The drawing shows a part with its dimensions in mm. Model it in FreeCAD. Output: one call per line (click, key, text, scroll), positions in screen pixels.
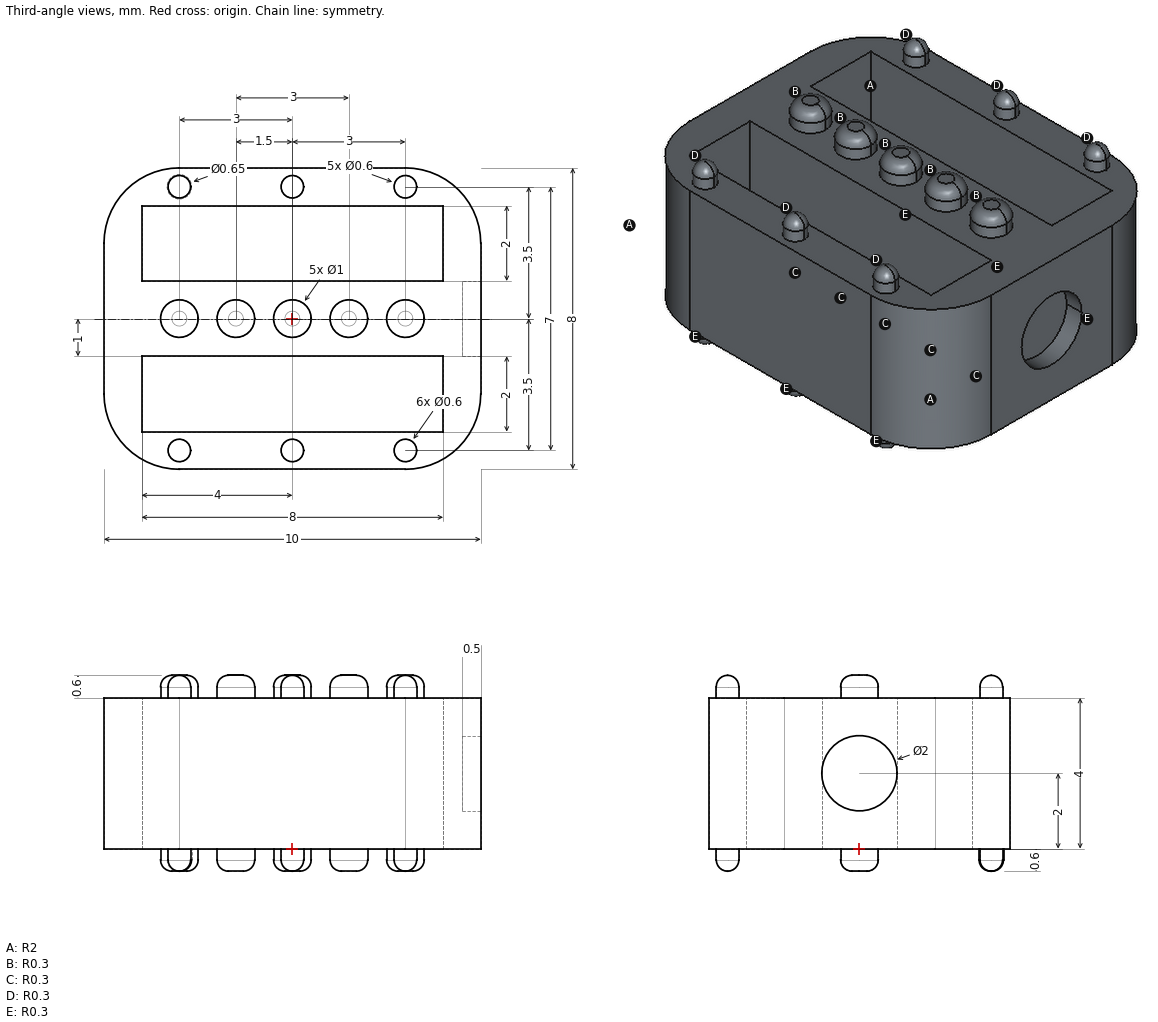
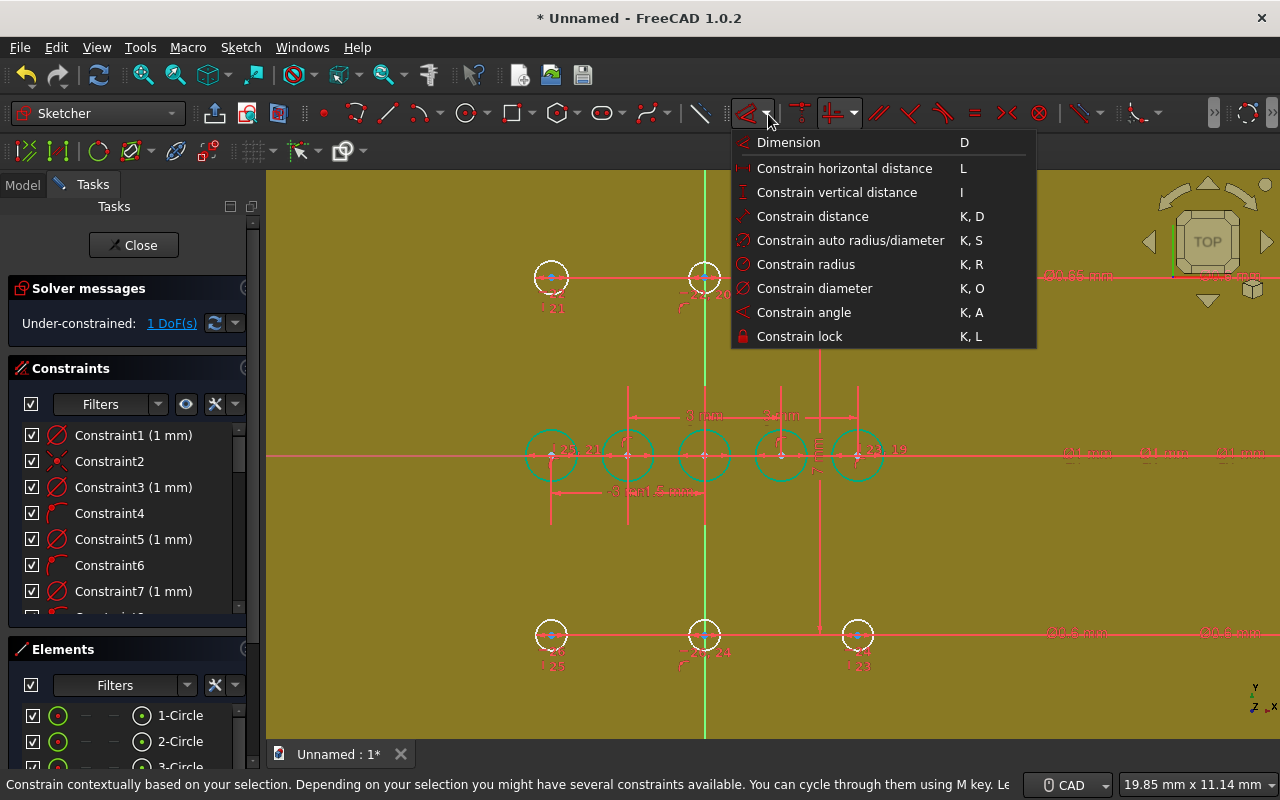
click(884, 192)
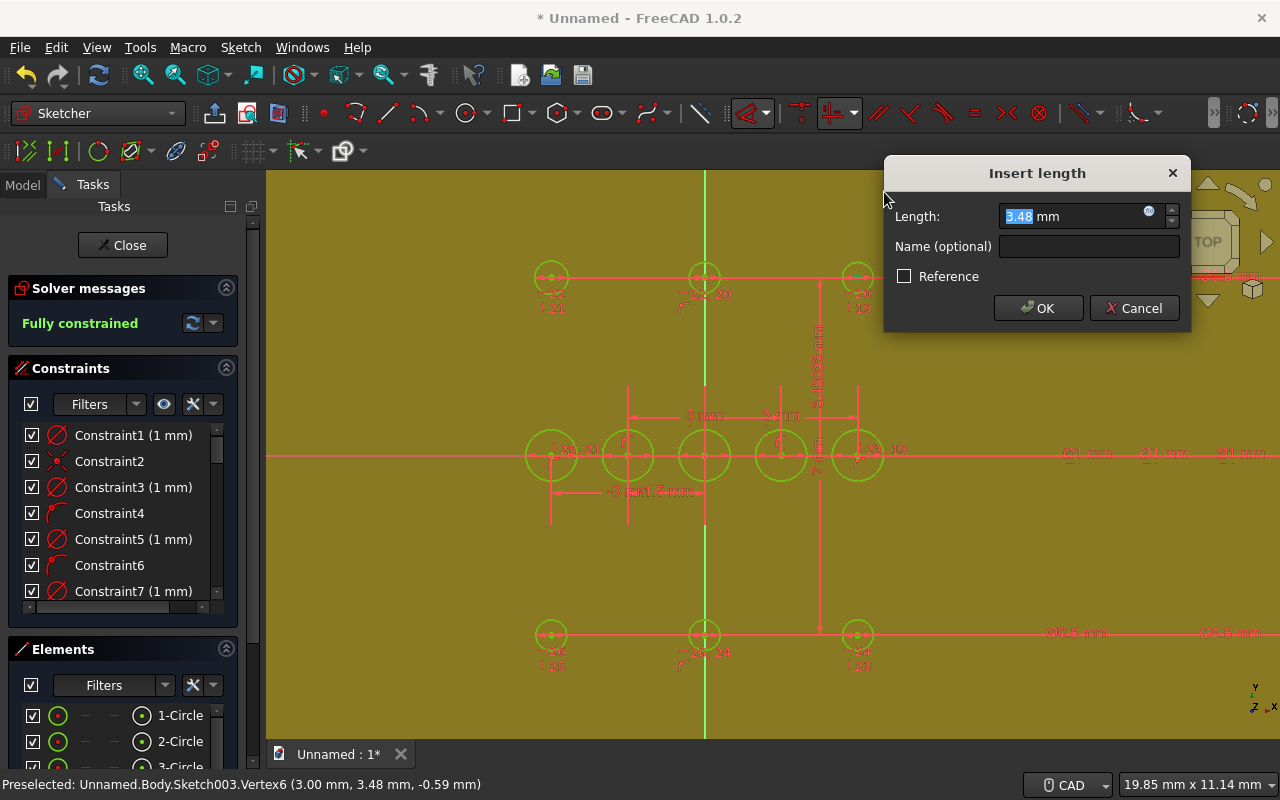
text(3.5)
key(Return)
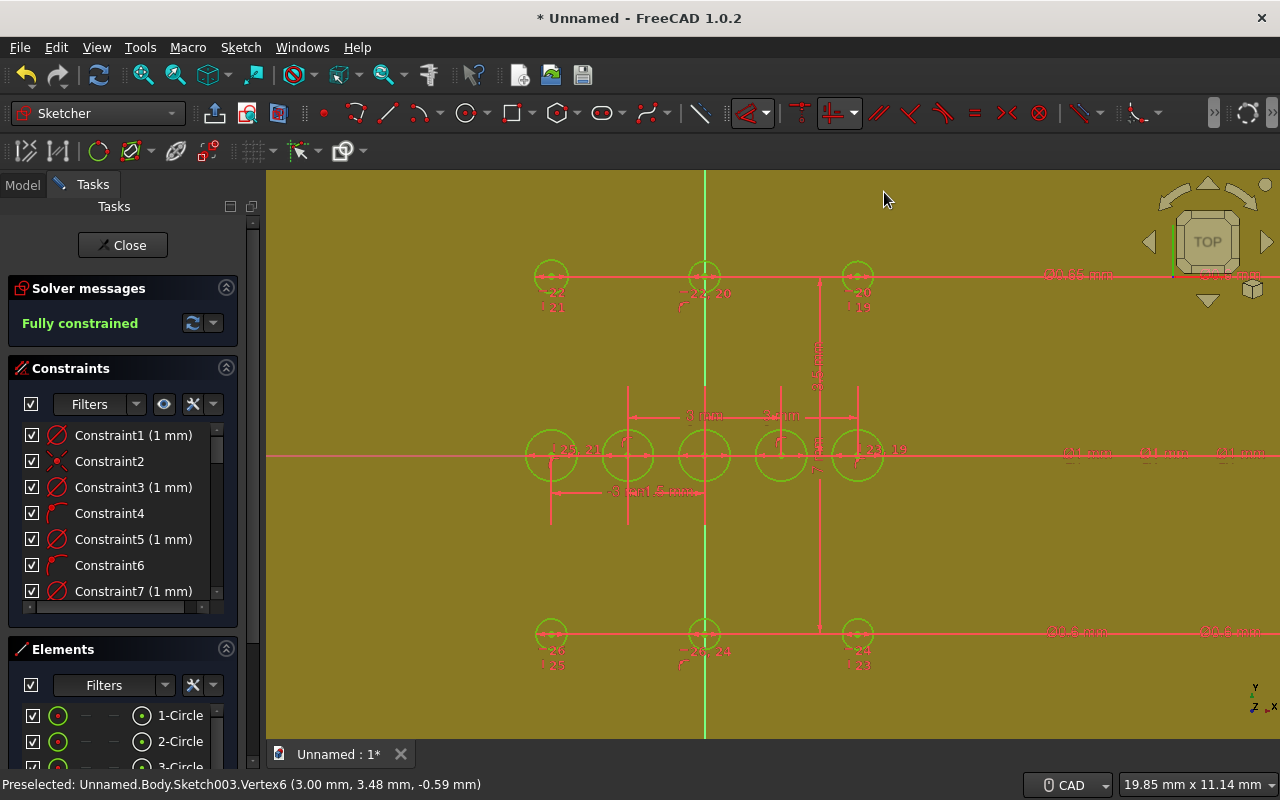
click(123, 245)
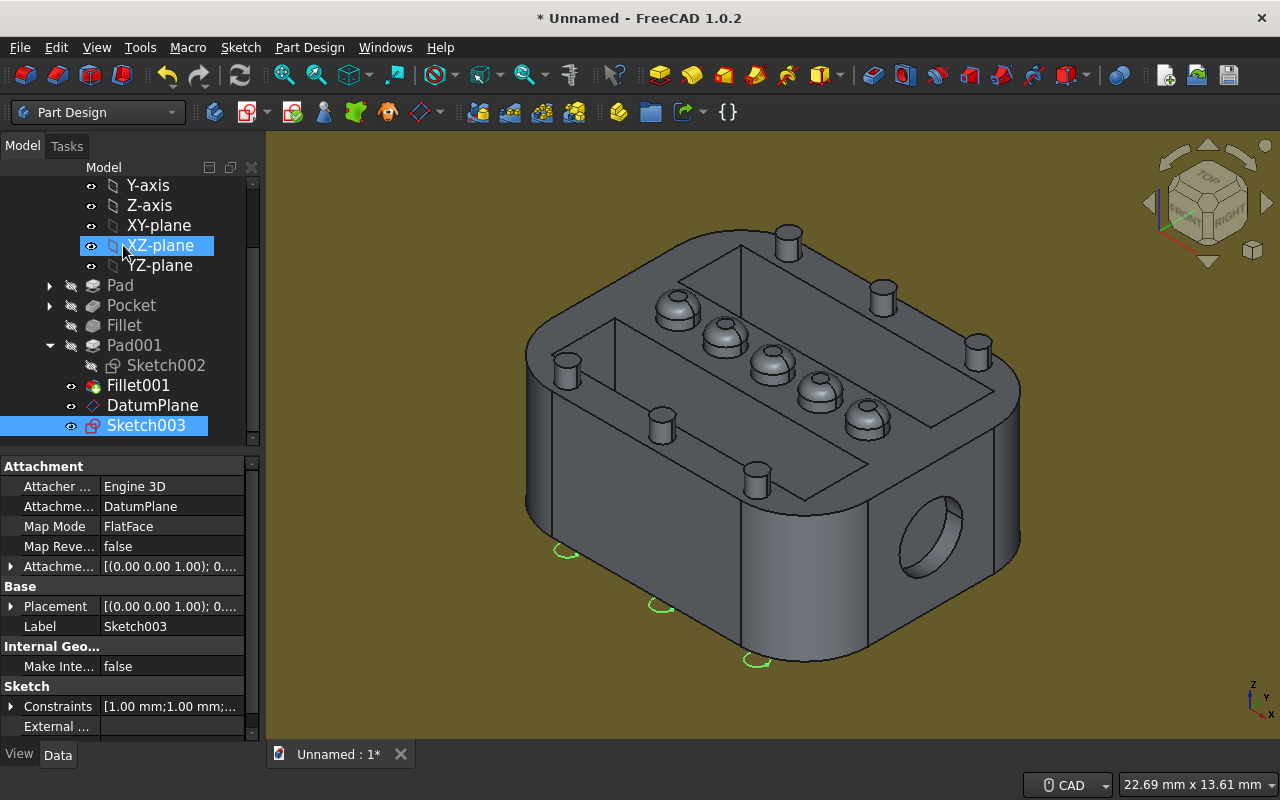
click(660, 76)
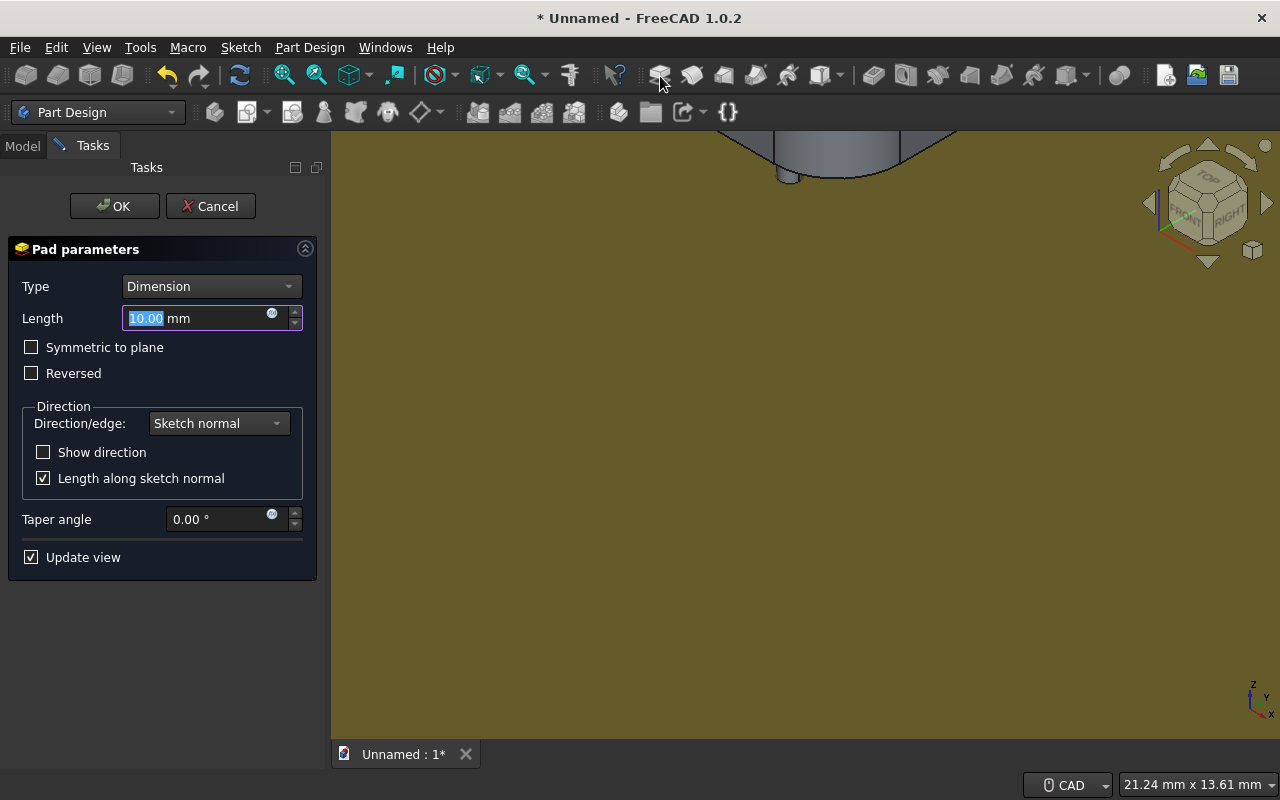
text(0.6)
key(Tab)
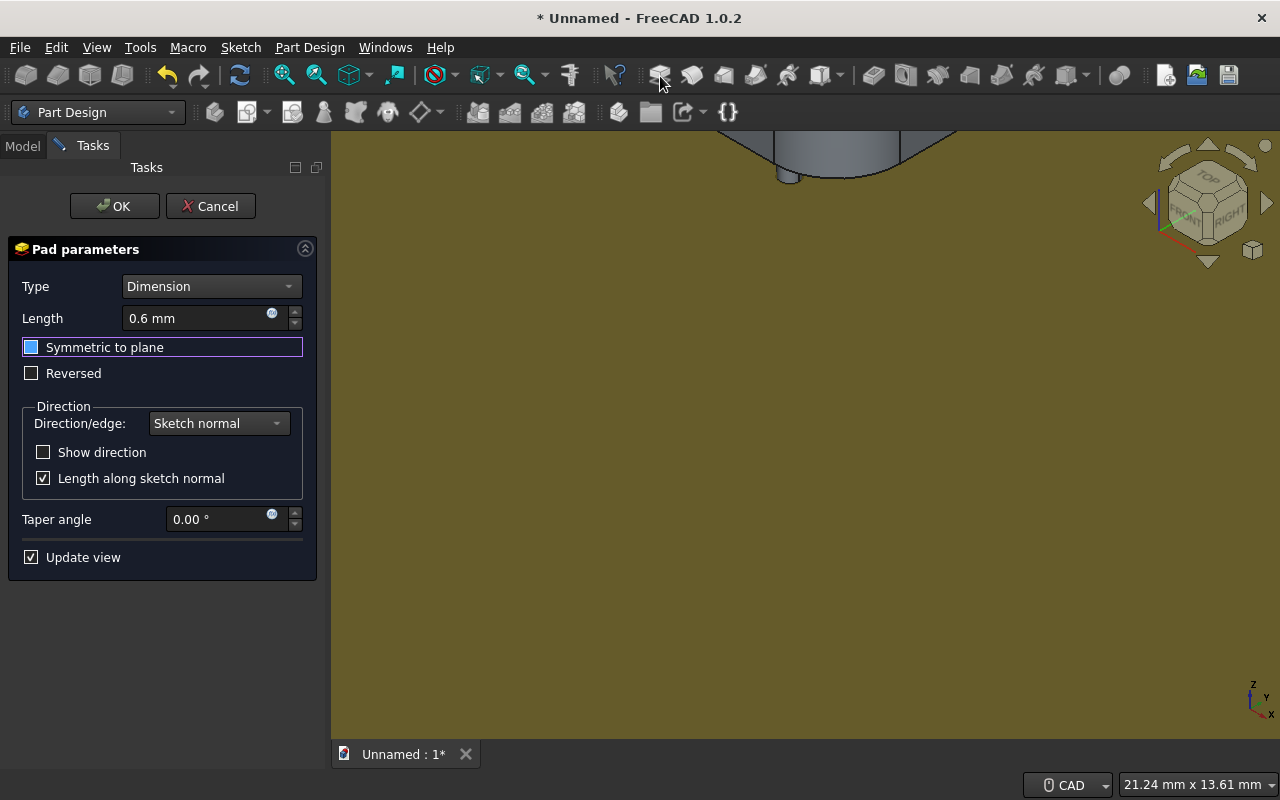
click(115, 206)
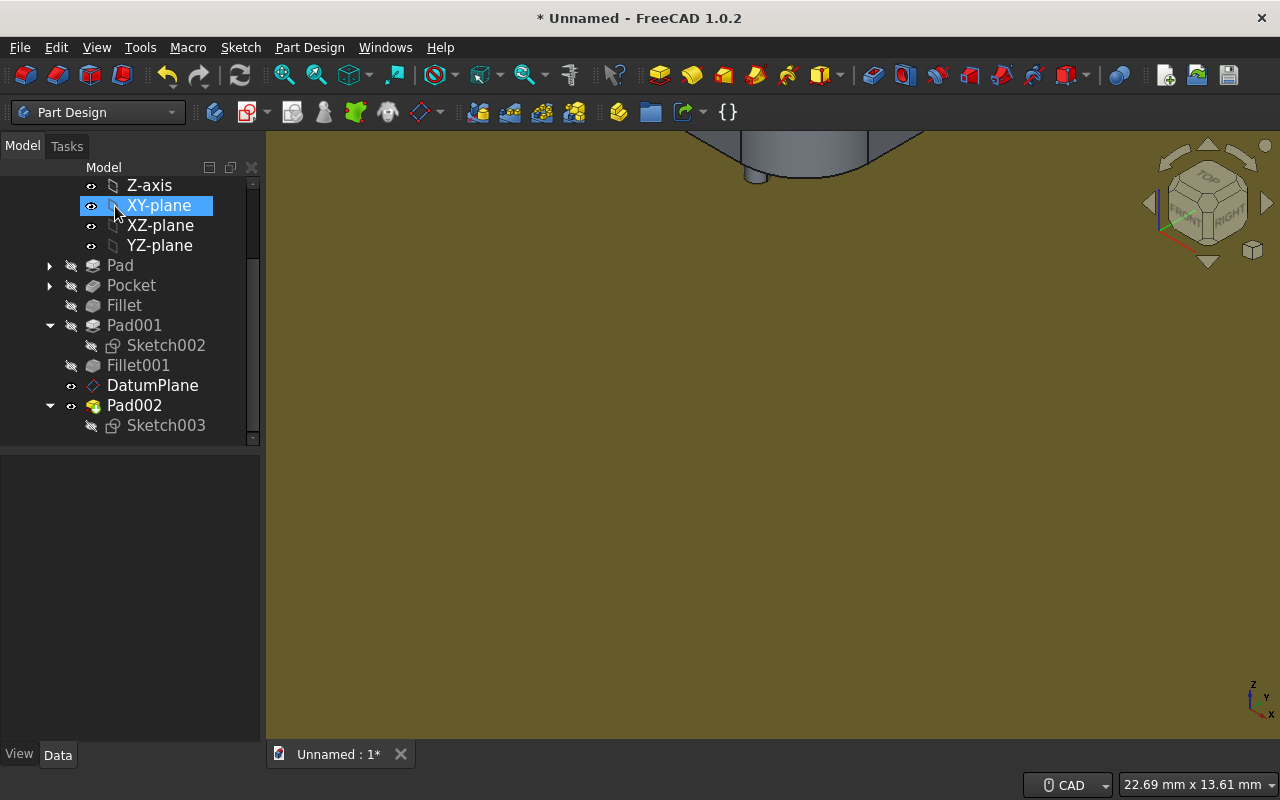
click(116, 386)
key(space)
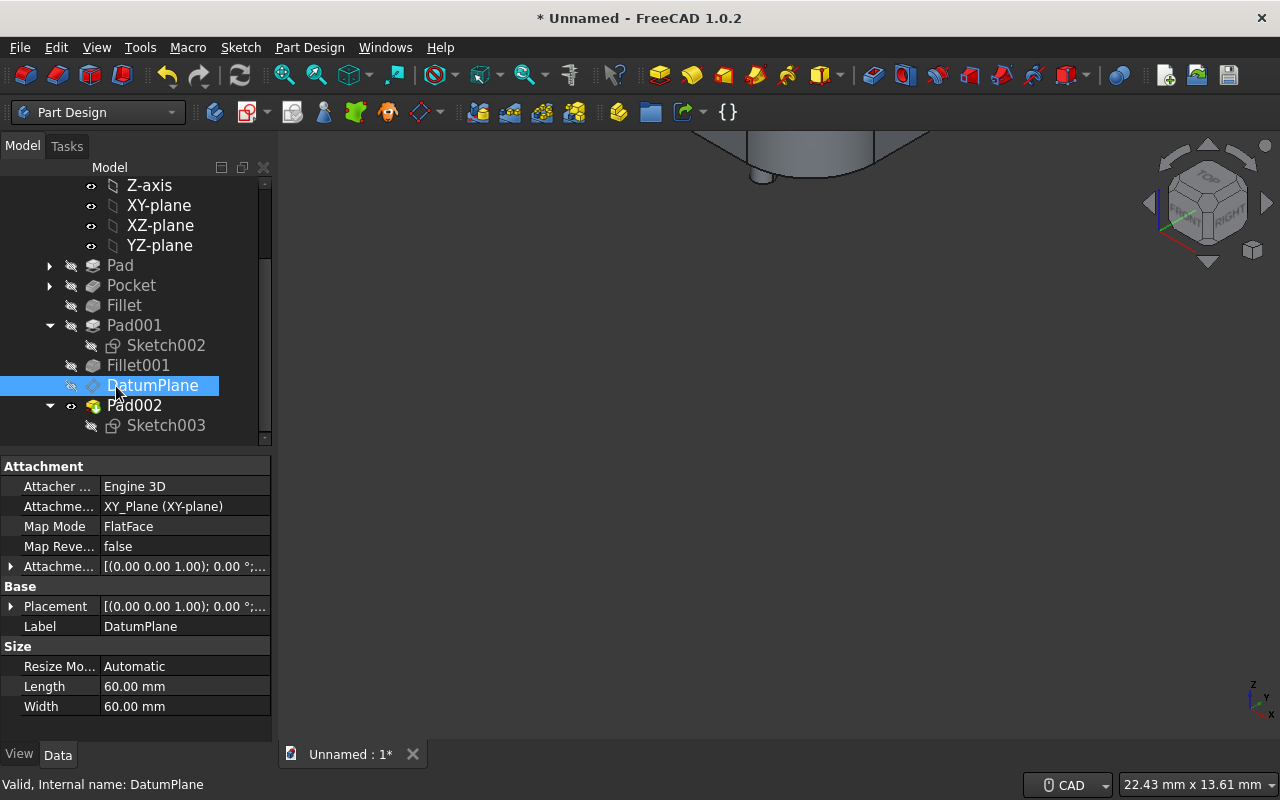
click(286, 76)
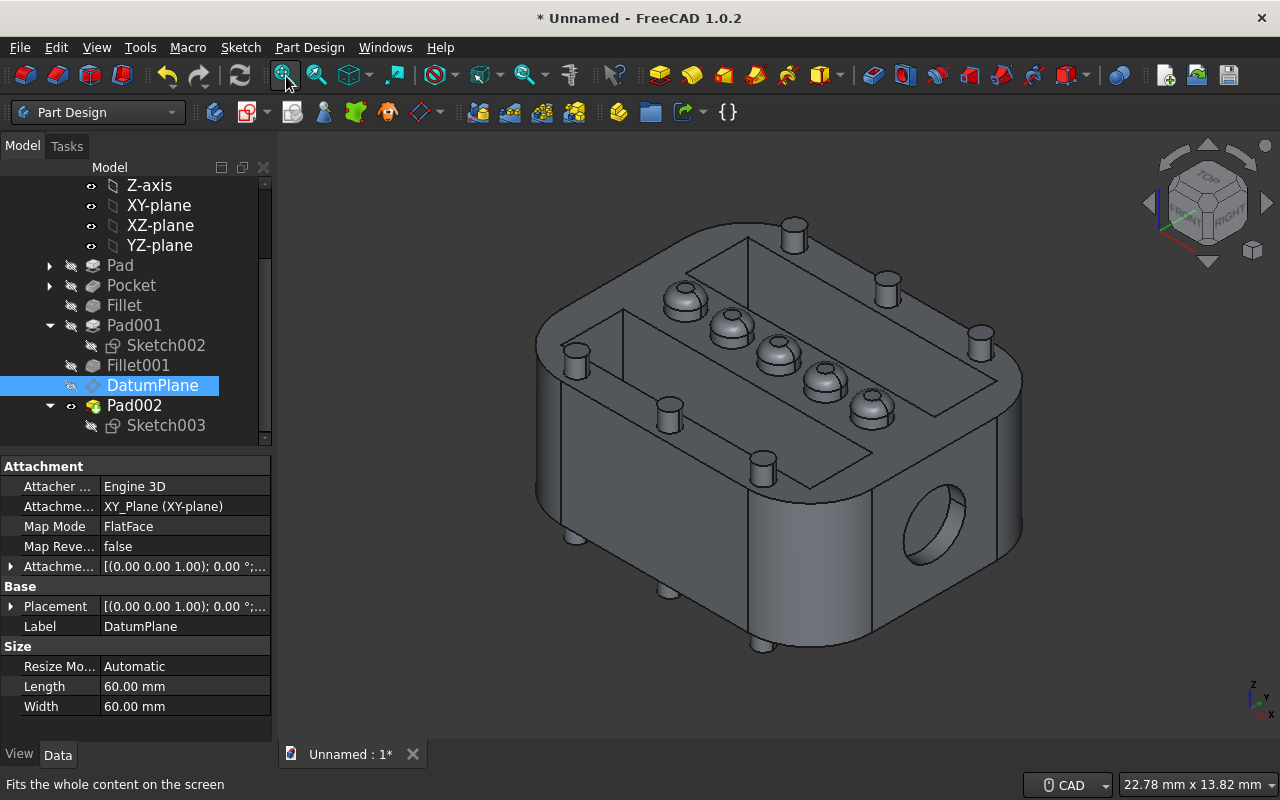
key(2)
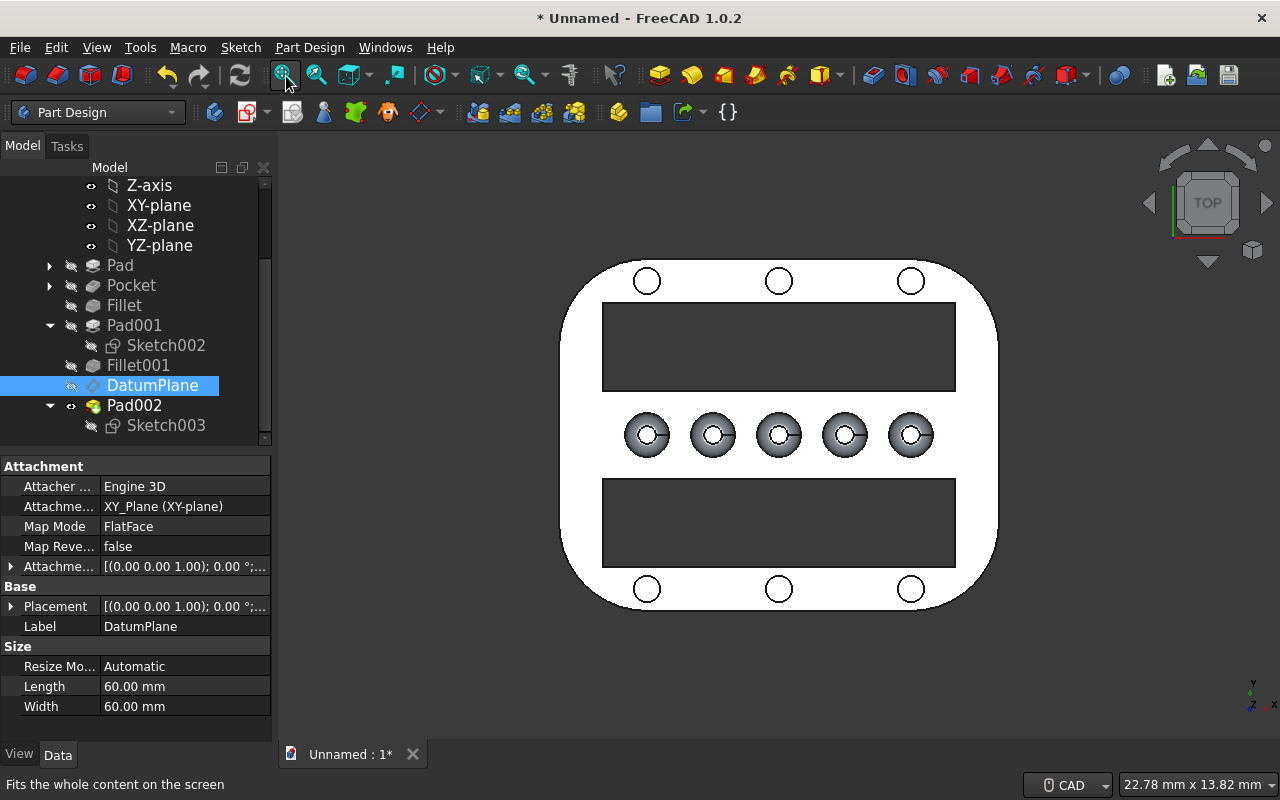
key(0)